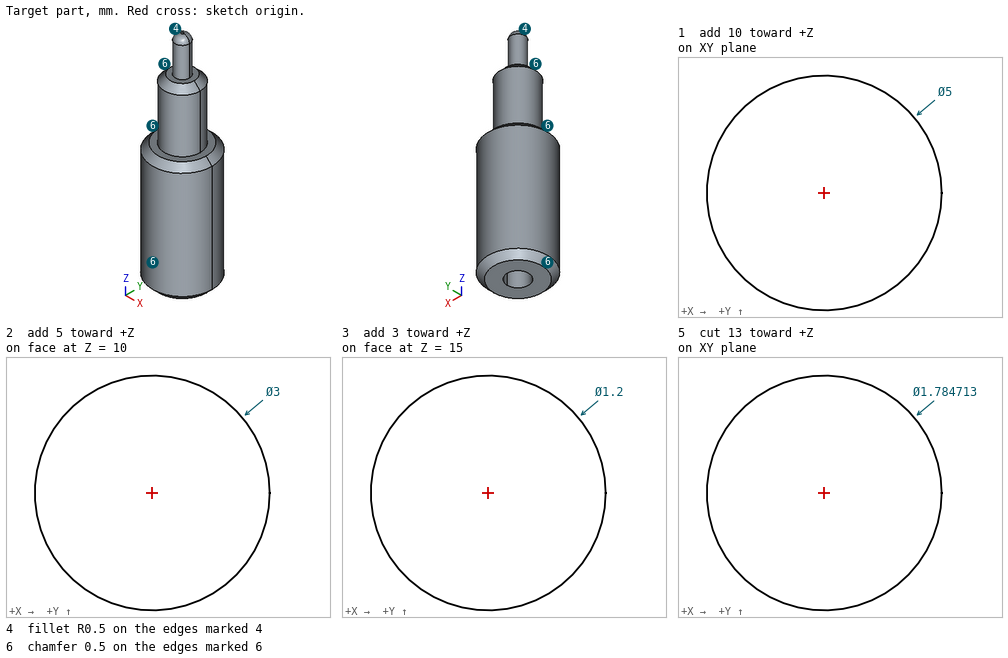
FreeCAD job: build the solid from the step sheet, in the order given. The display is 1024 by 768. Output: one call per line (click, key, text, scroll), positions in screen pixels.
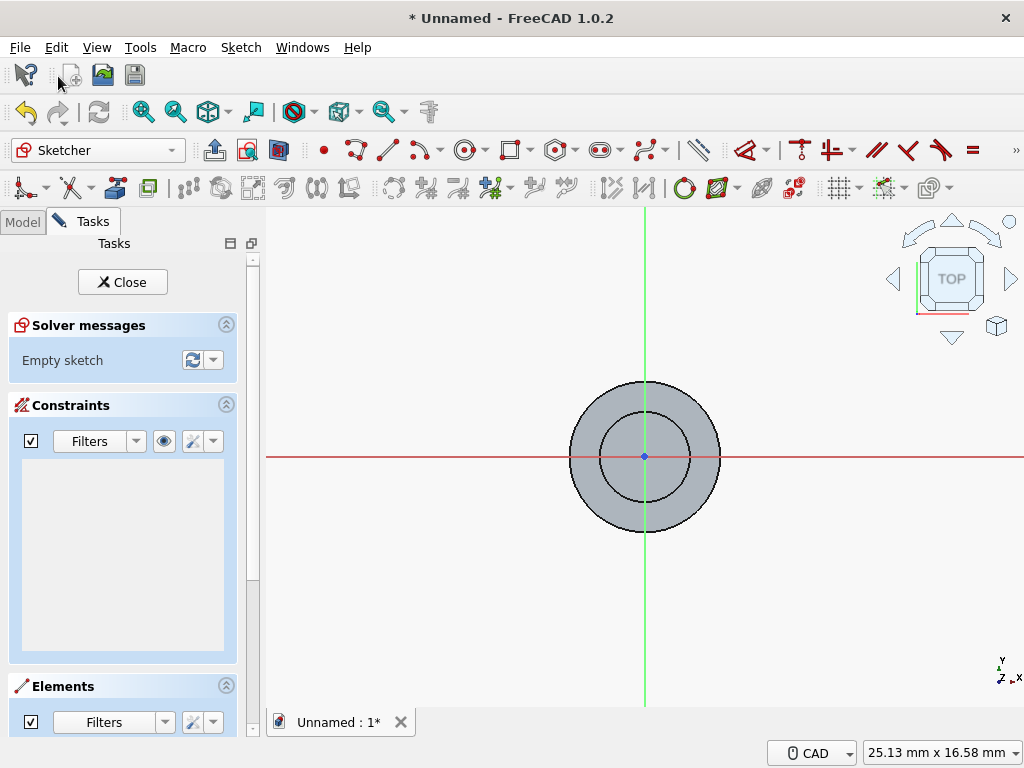
scroll(653, 457, up, 11)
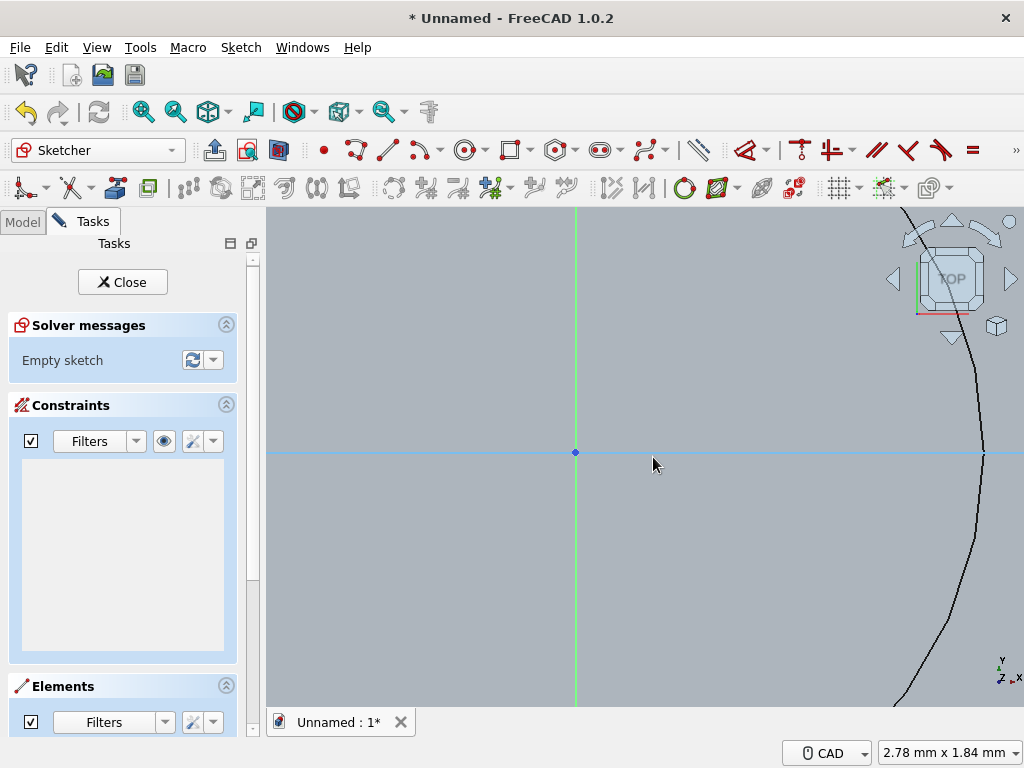
click(466, 150)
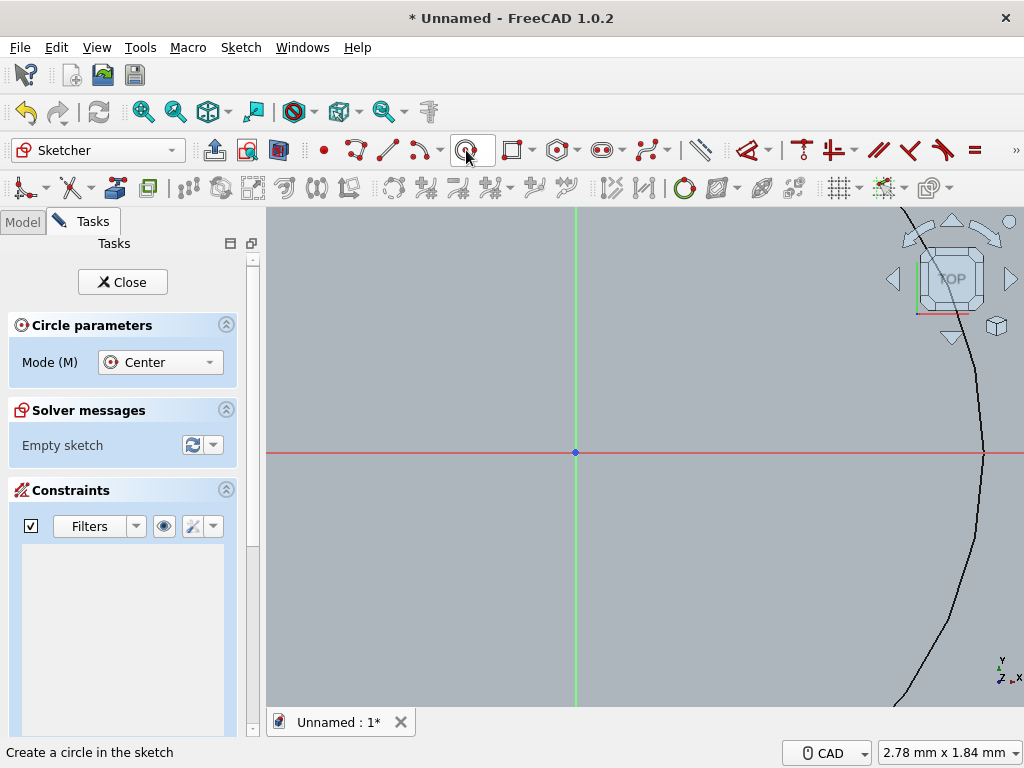
click(576, 453)
move(691, 338)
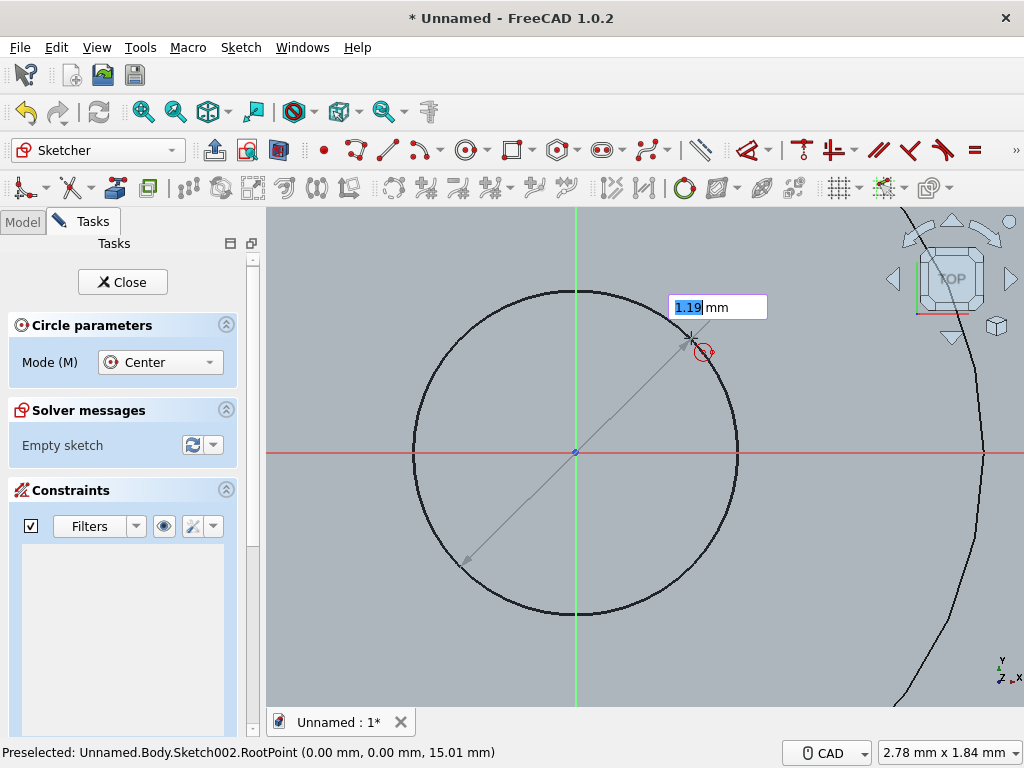
text(1.2)
key(Return)
key(Escape)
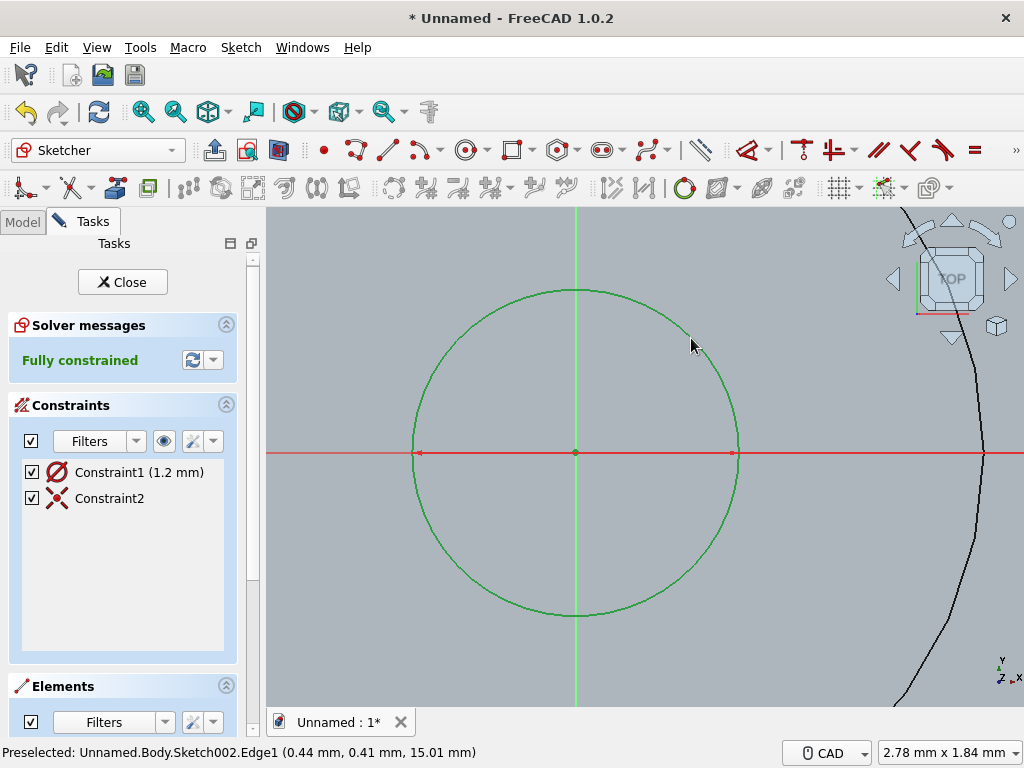
click(123, 282)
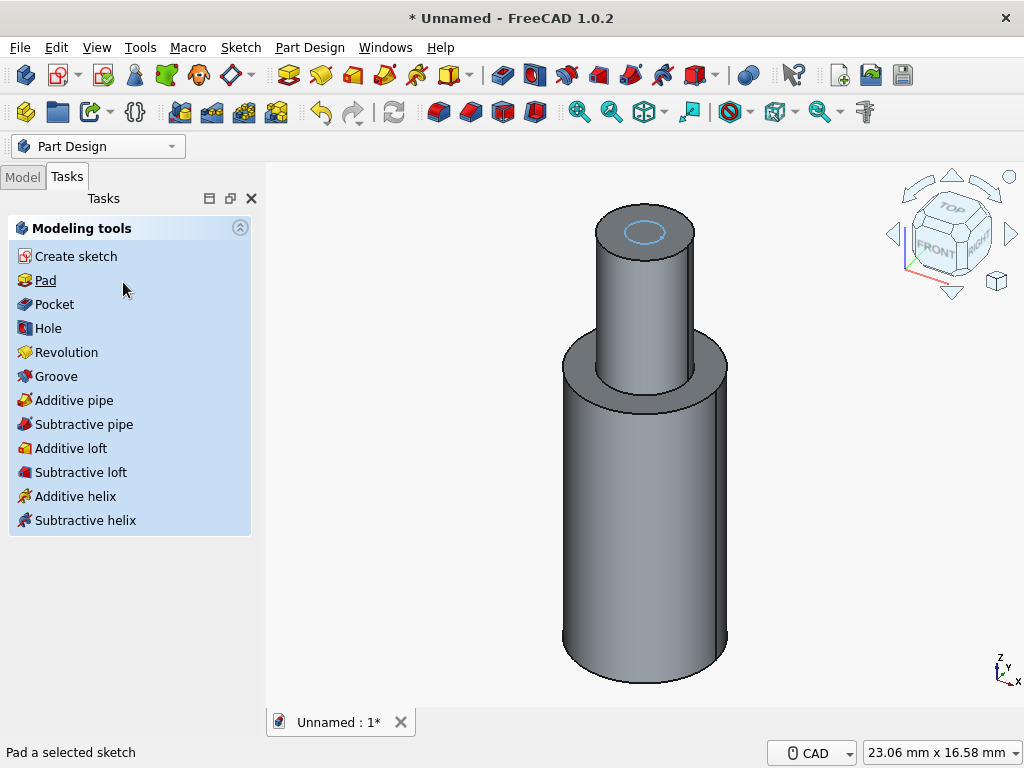
click(290, 76)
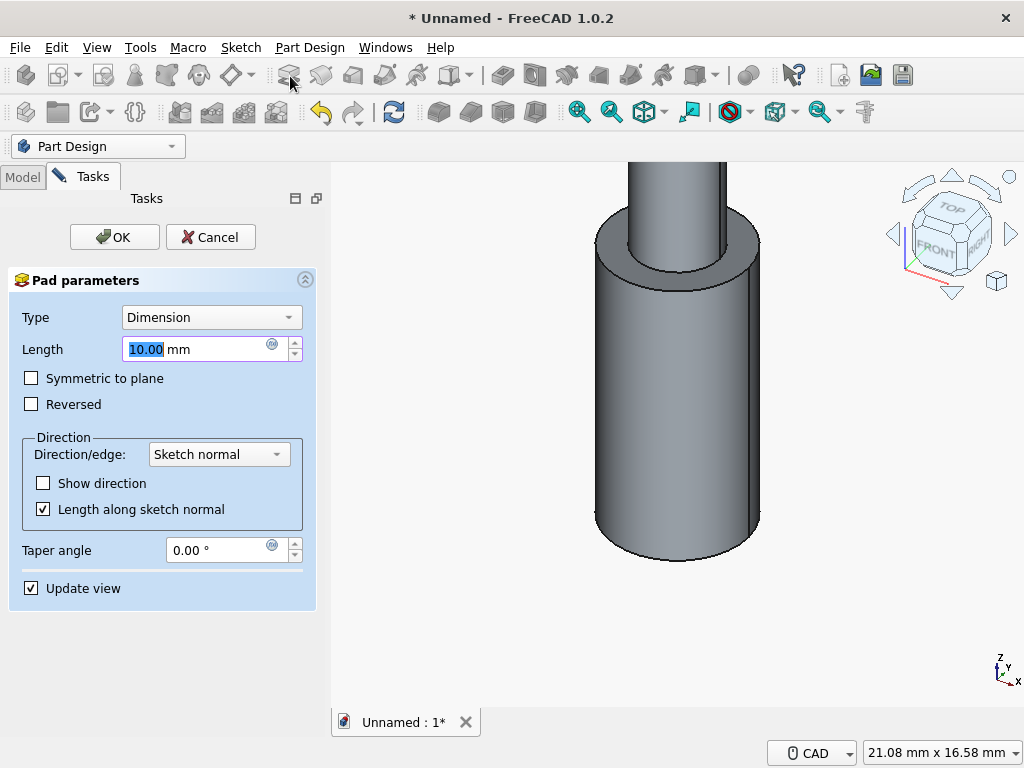
text(3)
key(Tab)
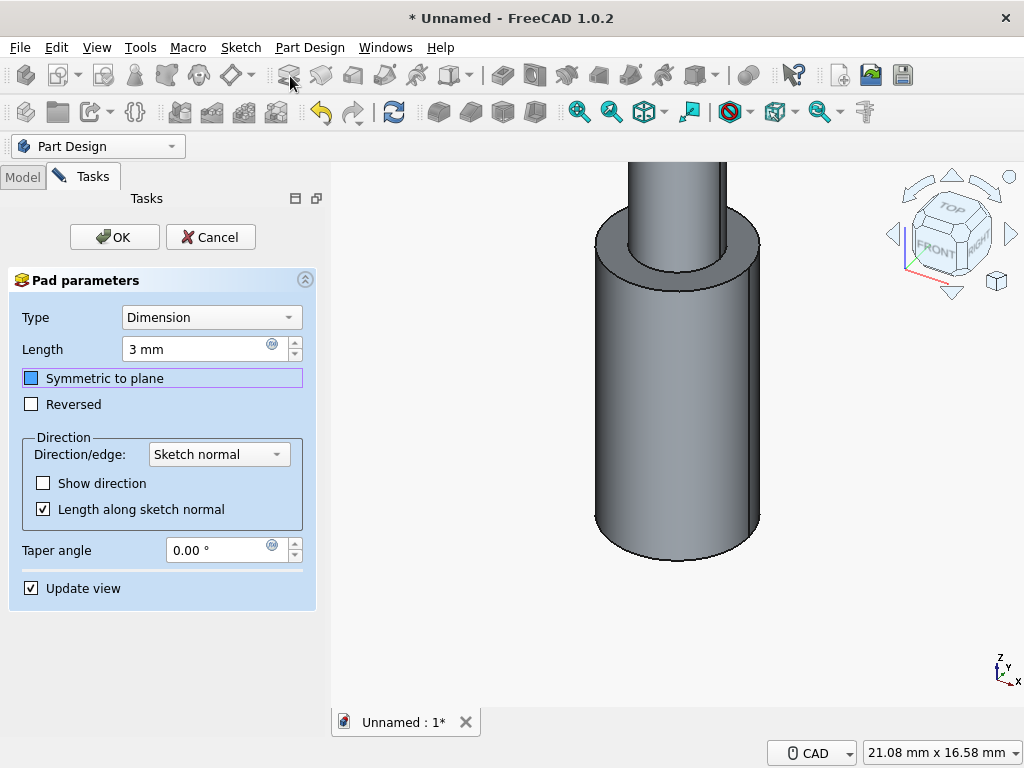
click(115, 237)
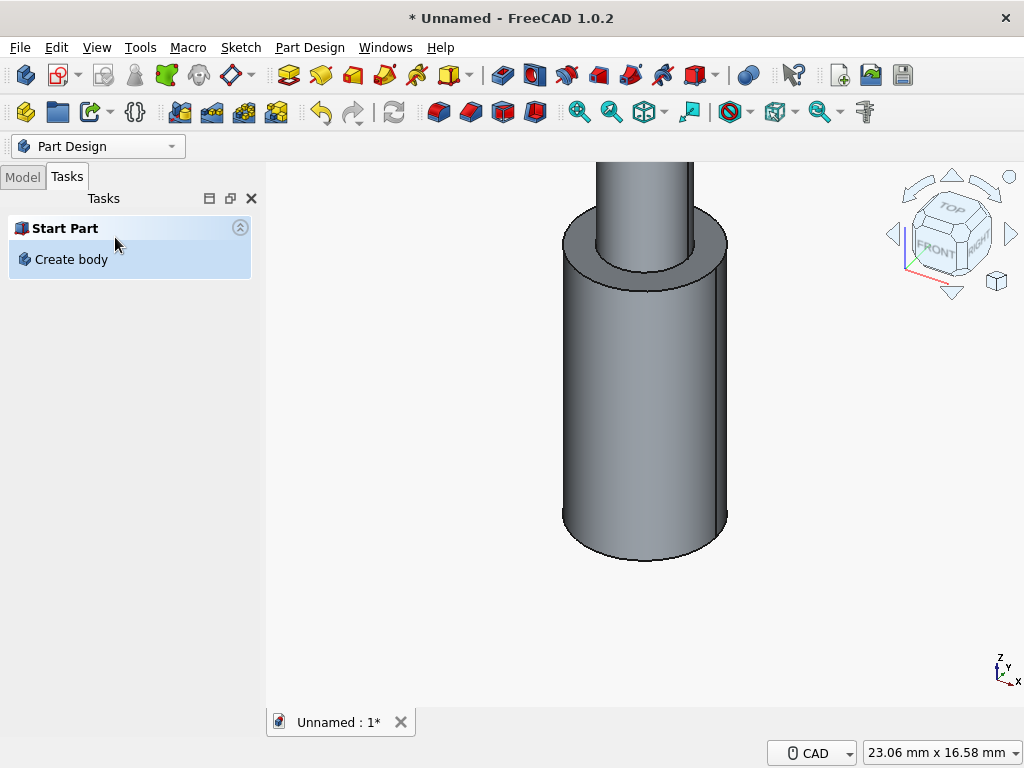
key(v)
key(f)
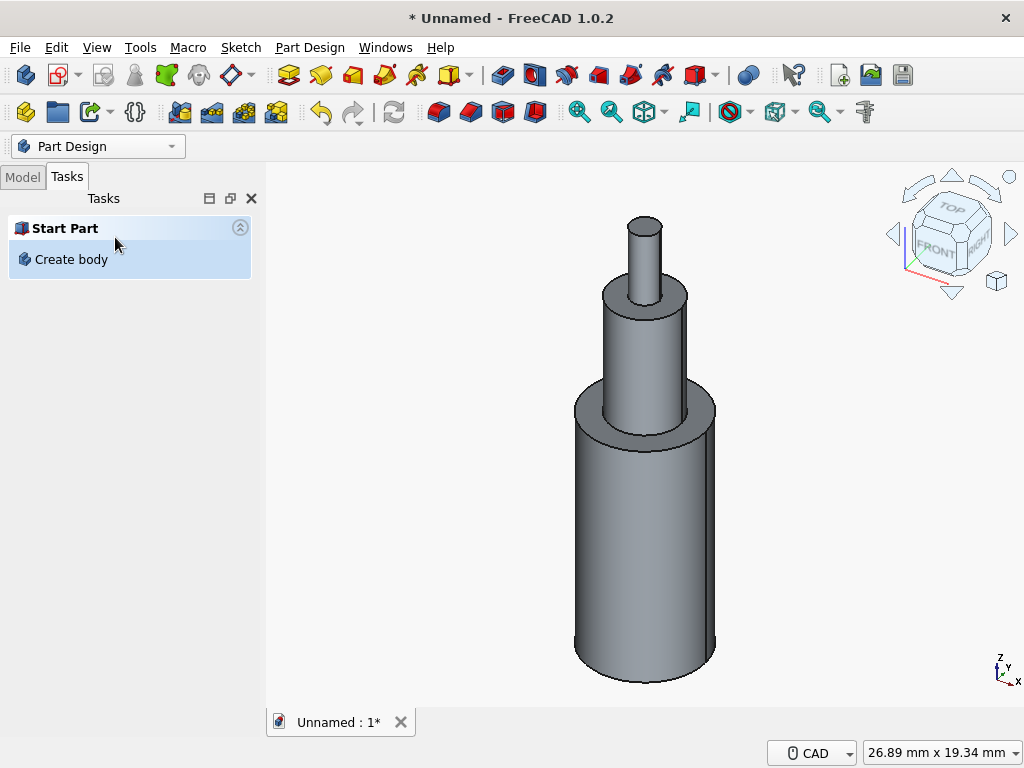
click(630, 221)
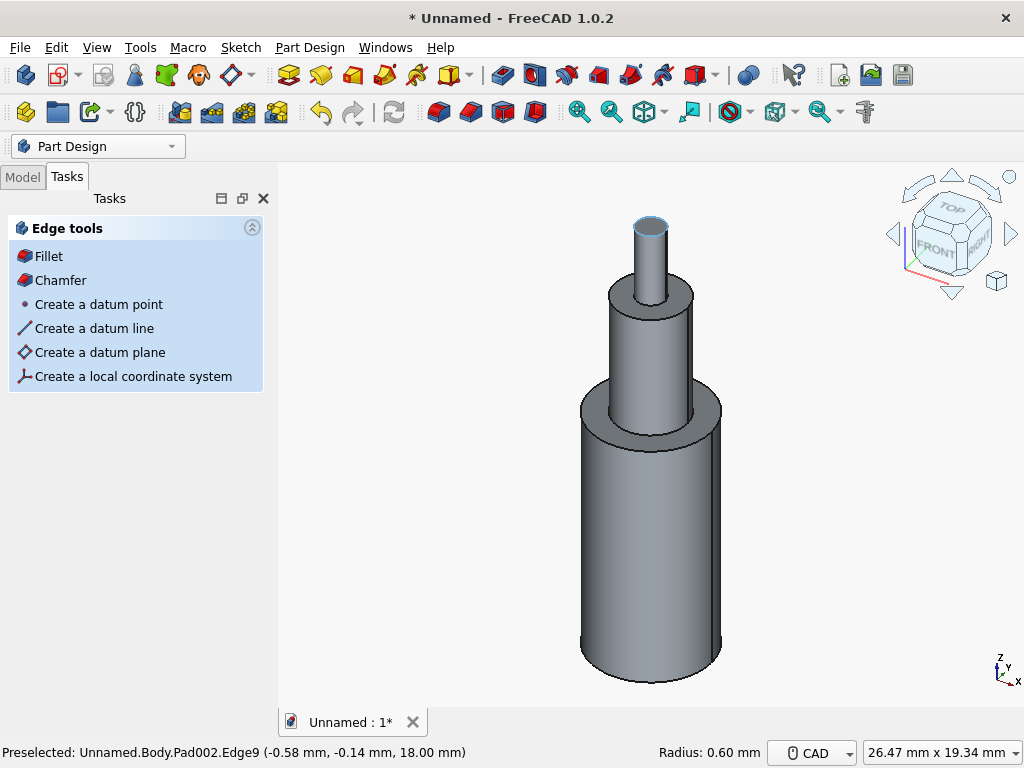
click(440, 112)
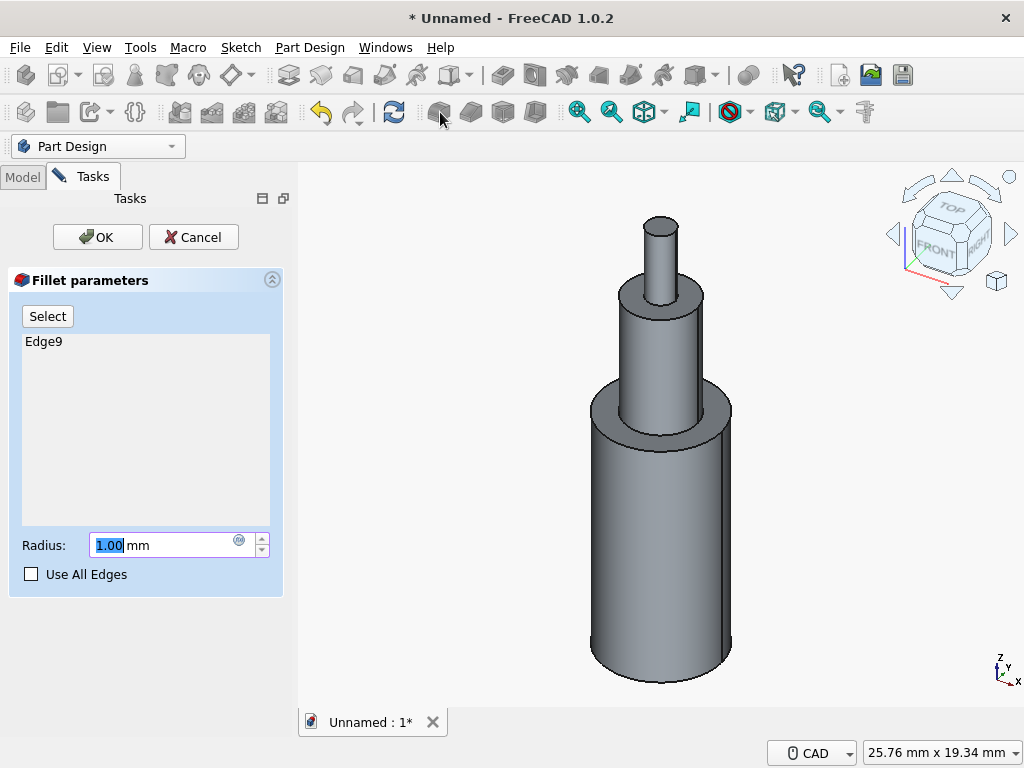
text(0.5)
key(Tab)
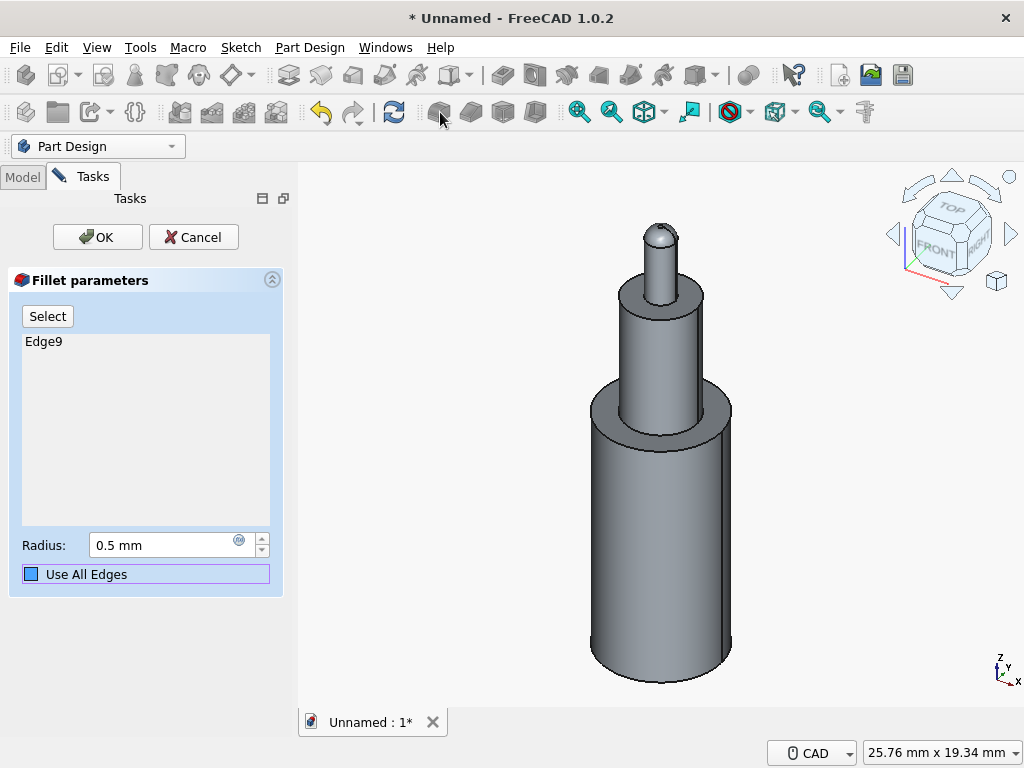
click(98, 237)